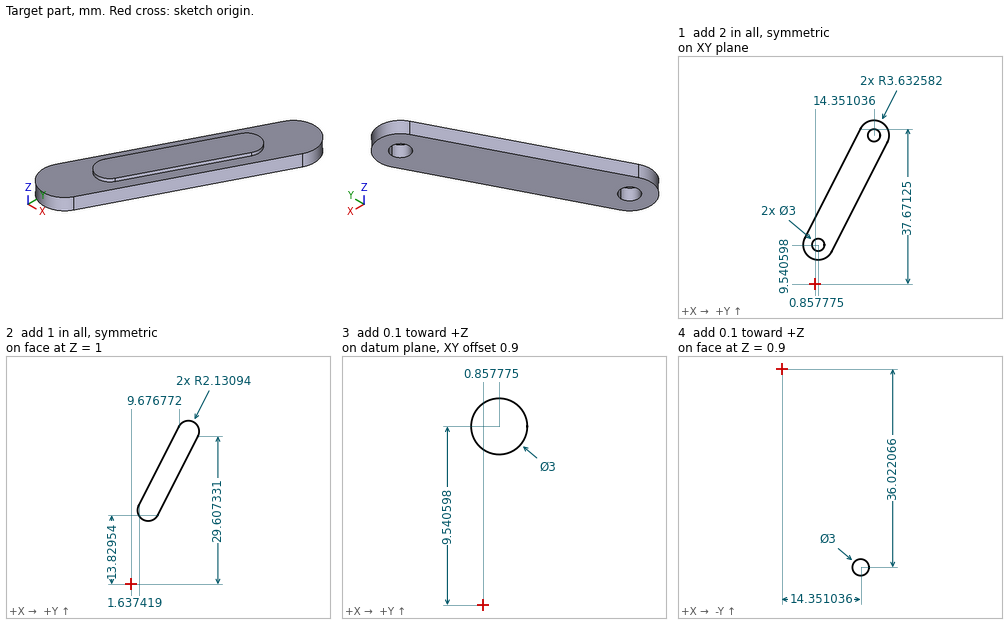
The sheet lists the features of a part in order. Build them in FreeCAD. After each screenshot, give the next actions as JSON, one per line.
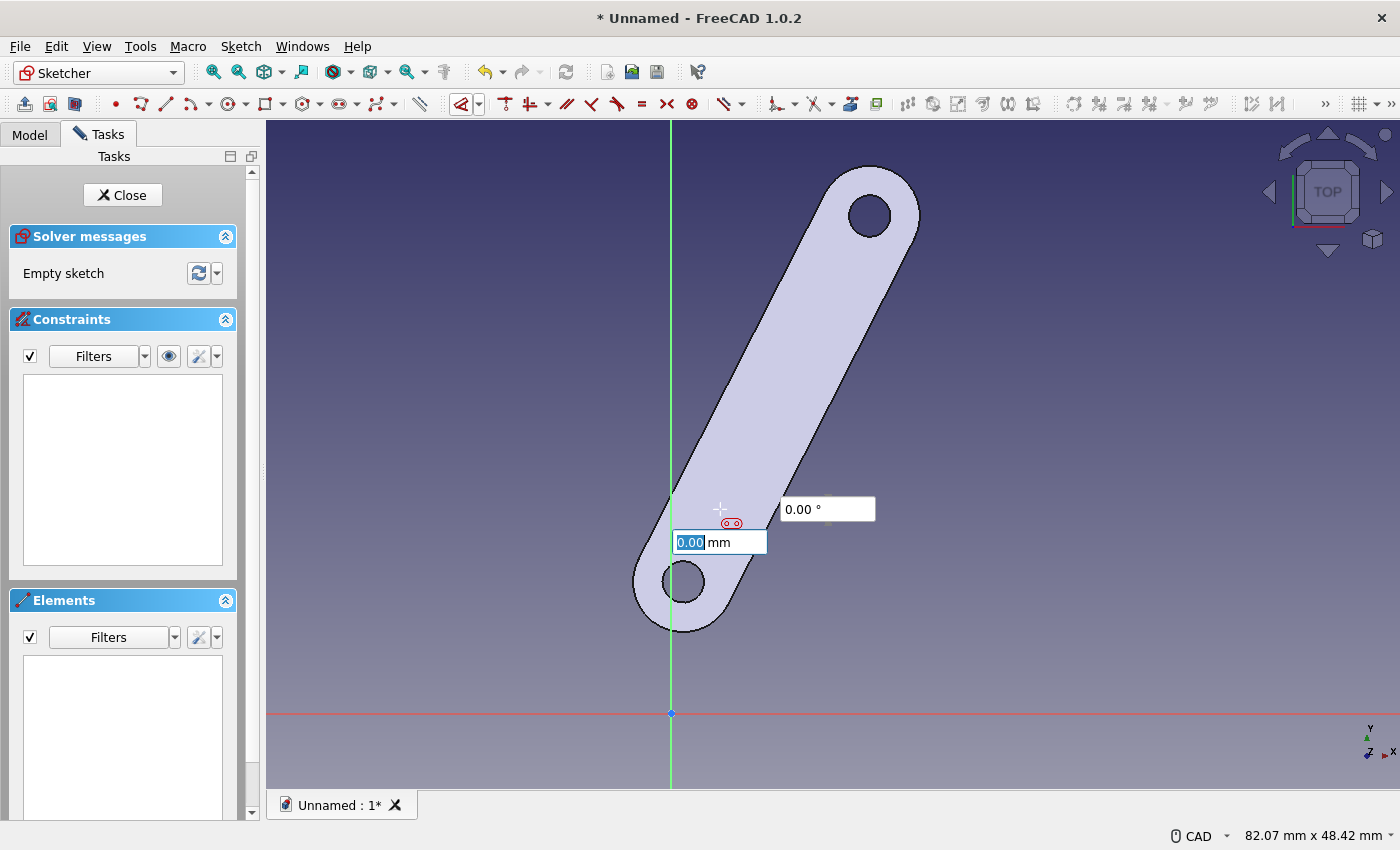
{"action": "left_click", "coordinate": [831, 291]}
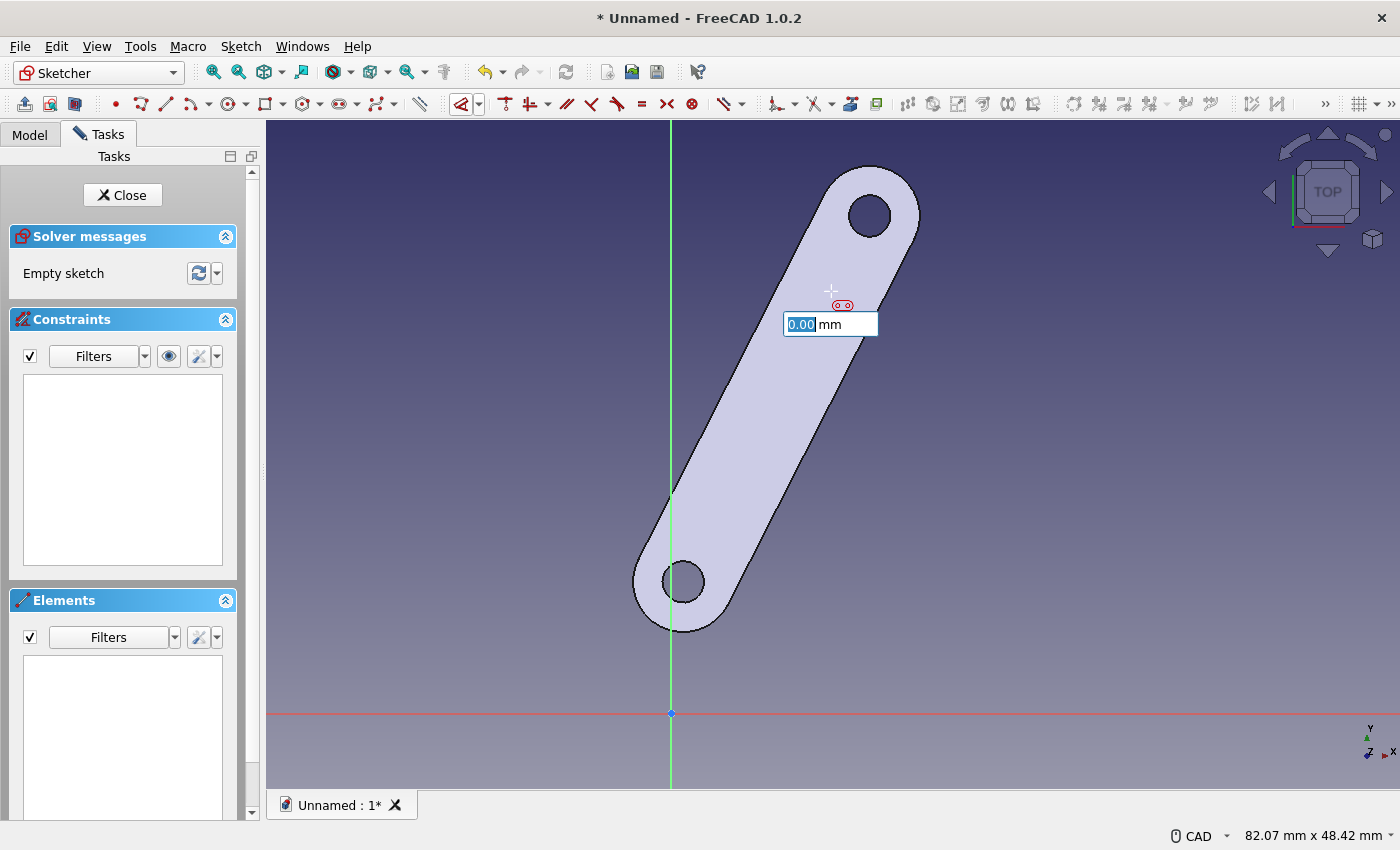
{"action": "left_click", "coordinate": [750, 387]}
{"action": "key", "text": "Escape"}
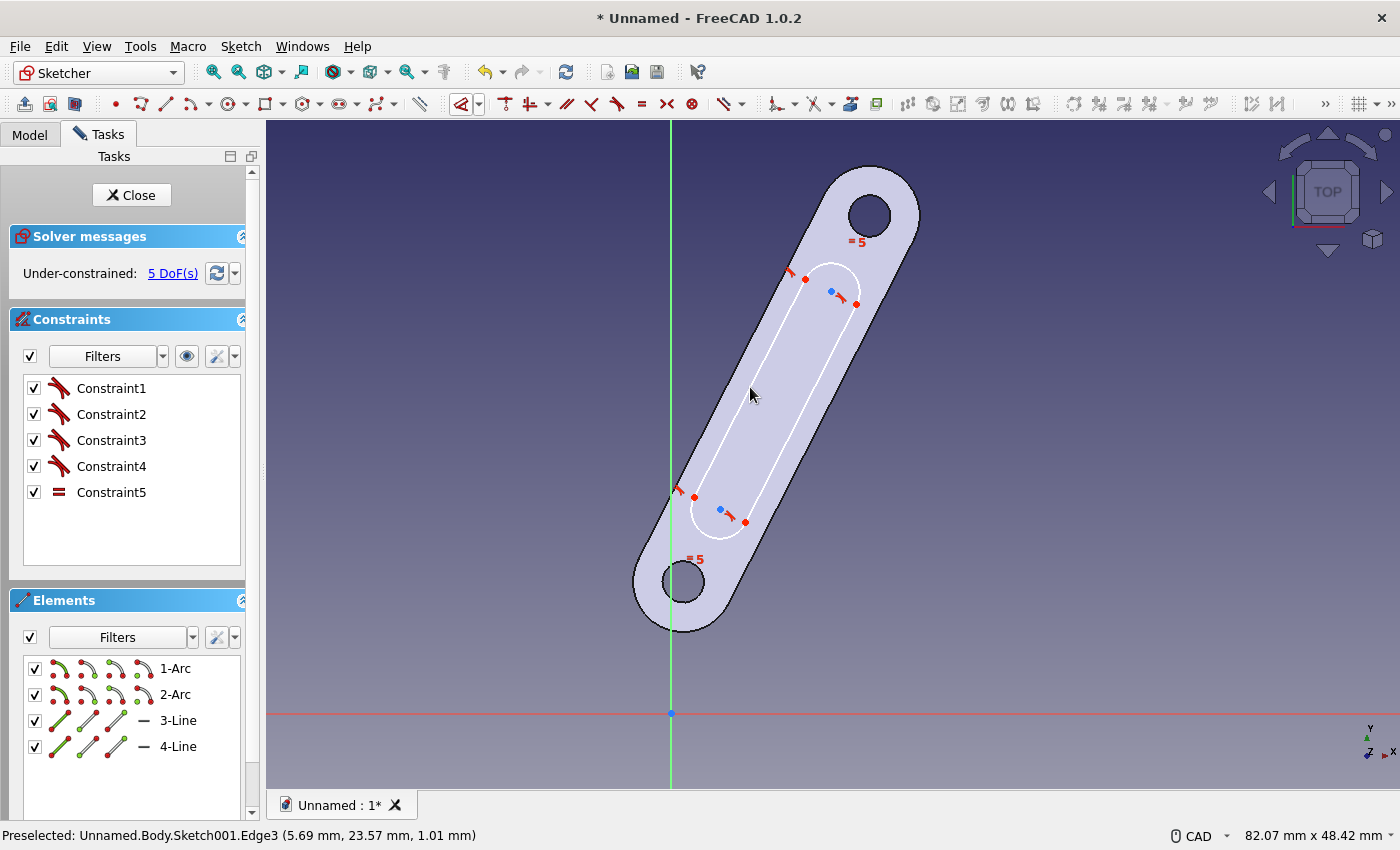
{"action": "scroll", "coordinate": [695, 523], "scroll_direction": "up", "scroll_amount": 2}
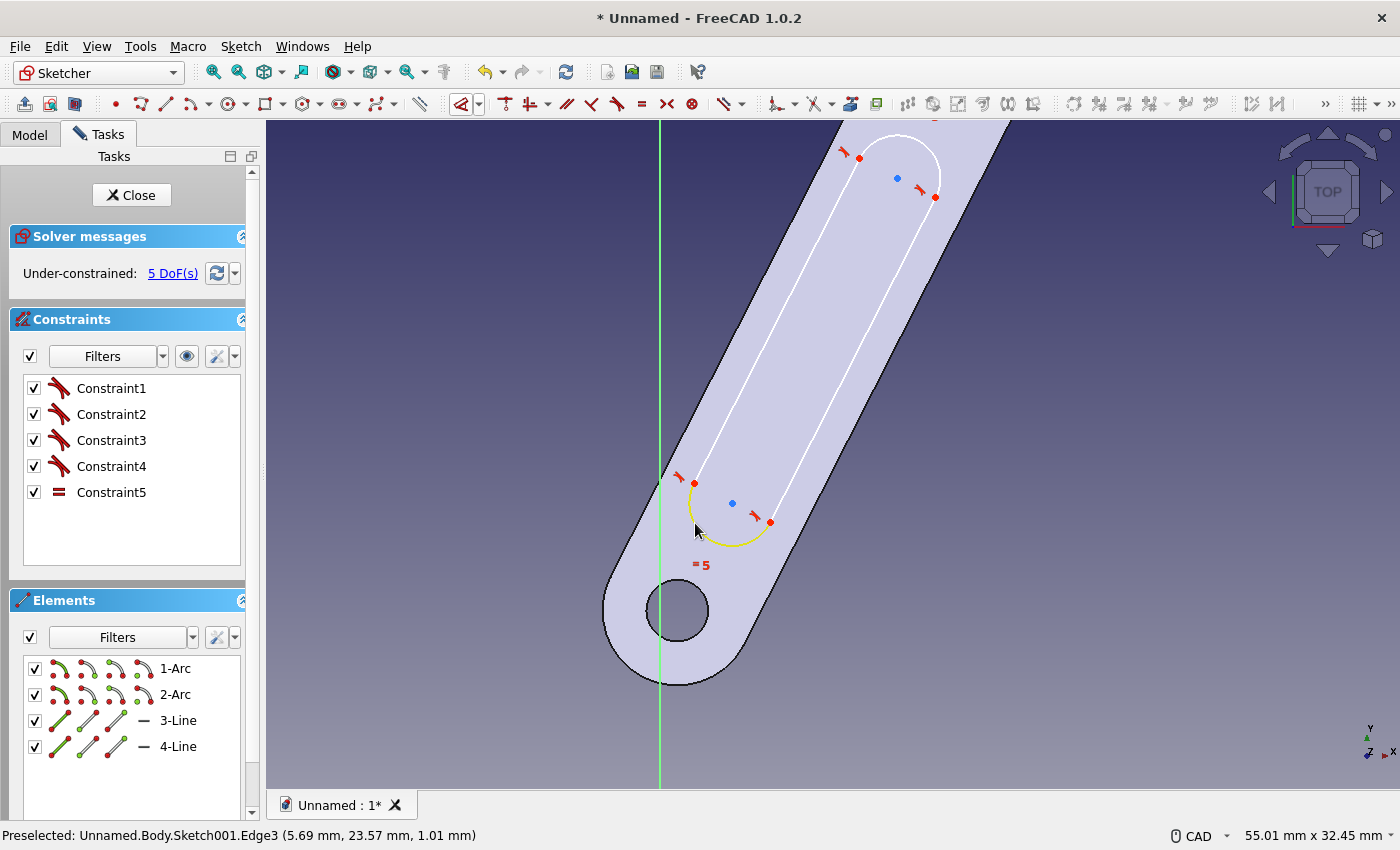
{"action": "left_click", "coordinate": [694, 523]}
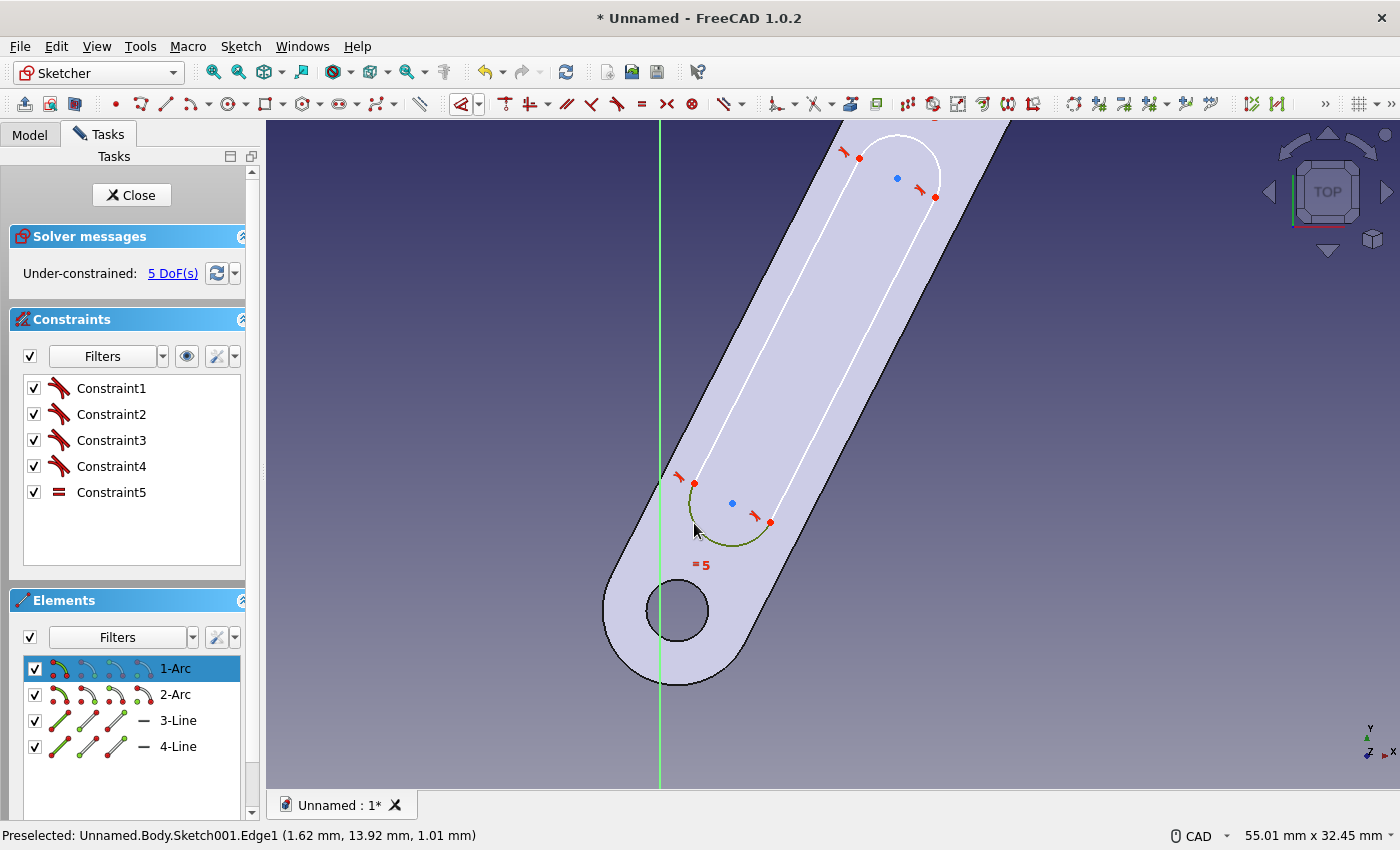
{"action": "left_click", "coordinate": [478, 104]}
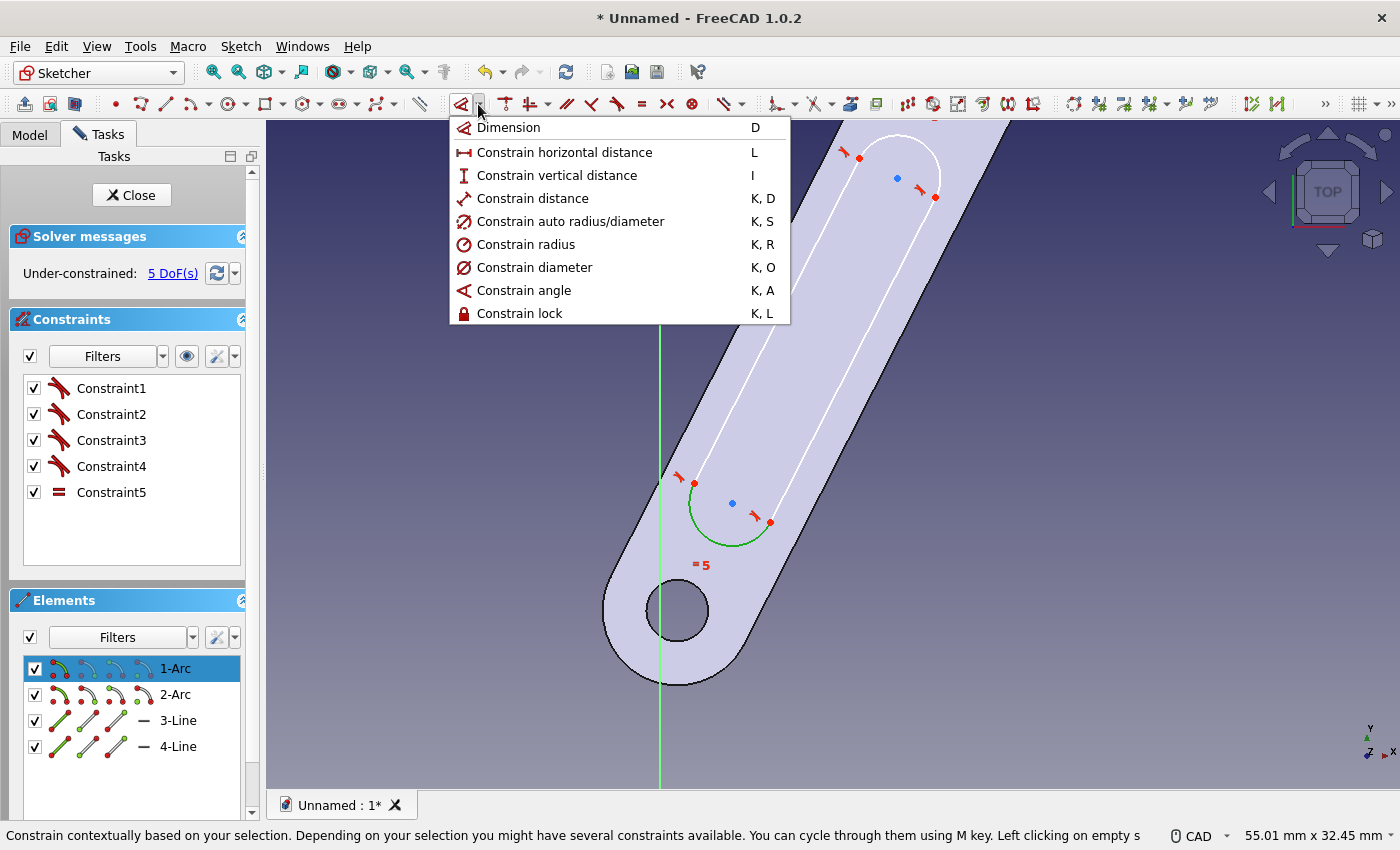
{"action": "left_click", "coordinate": [620, 244]}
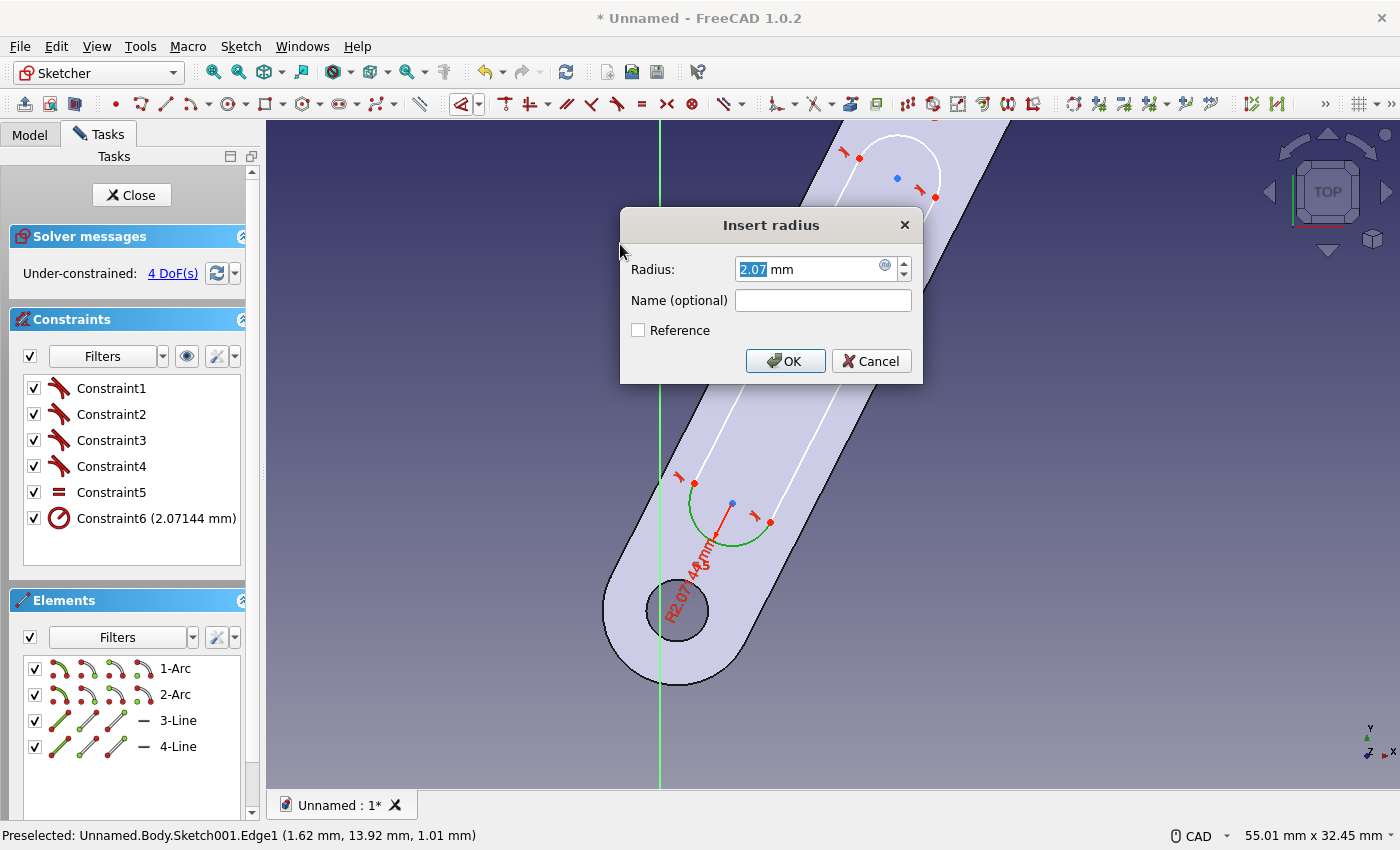
{"action": "type", "text": "2.13094"}
{"action": "key", "text": "Return"}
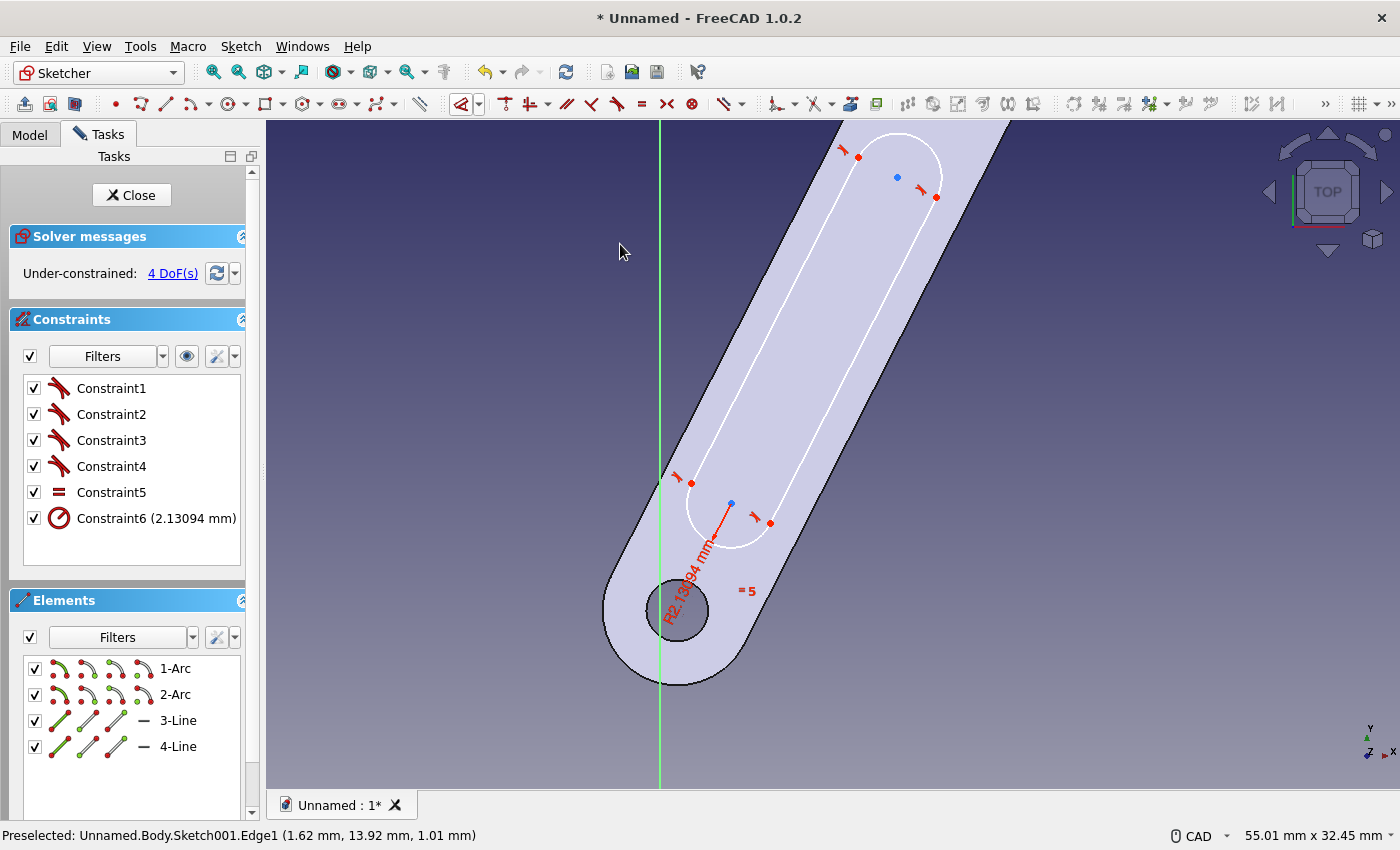
{"action": "left_click", "coordinate": [692, 484]}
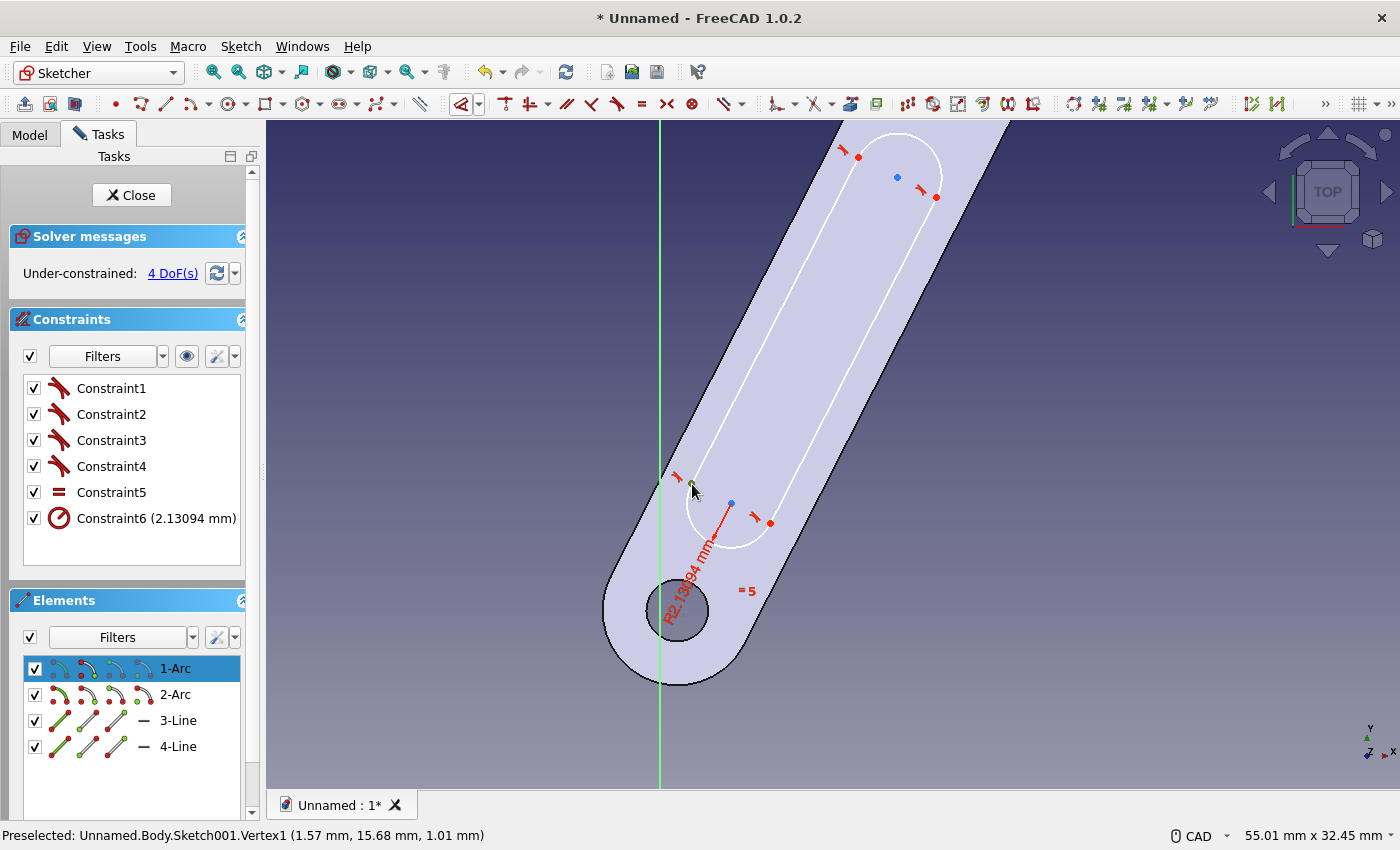
{"action": "left_click", "coordinate": [478, 104]}